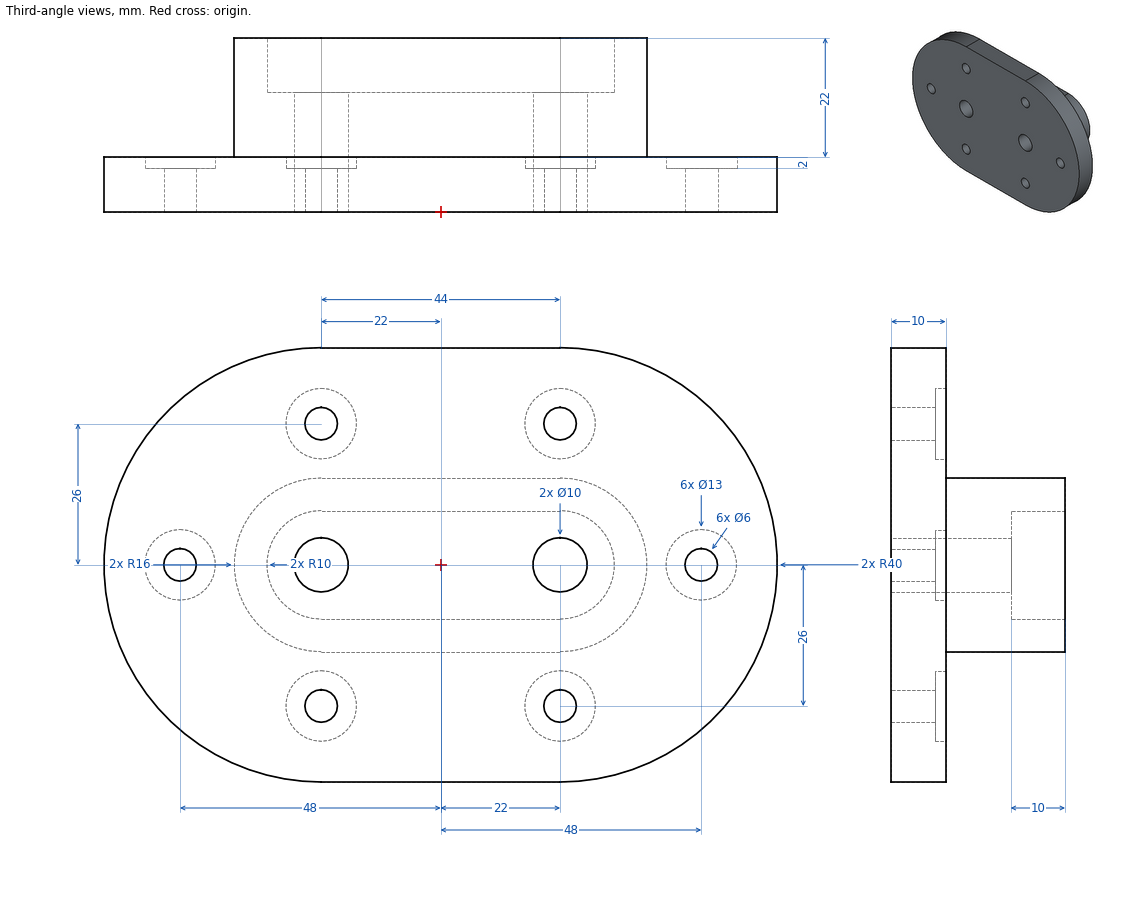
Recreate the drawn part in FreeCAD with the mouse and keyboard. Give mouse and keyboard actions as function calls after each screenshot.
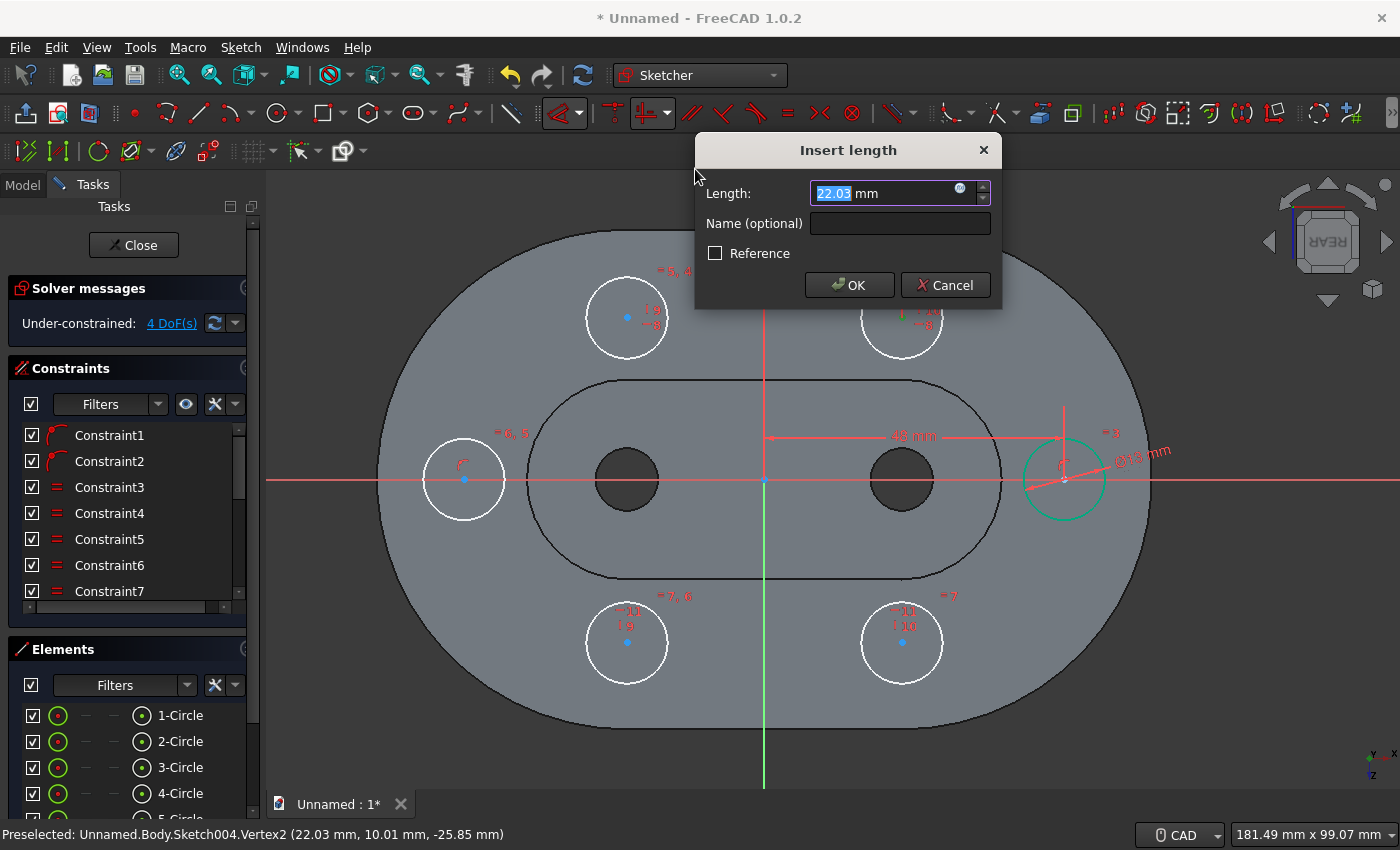
text(22)
key(Return)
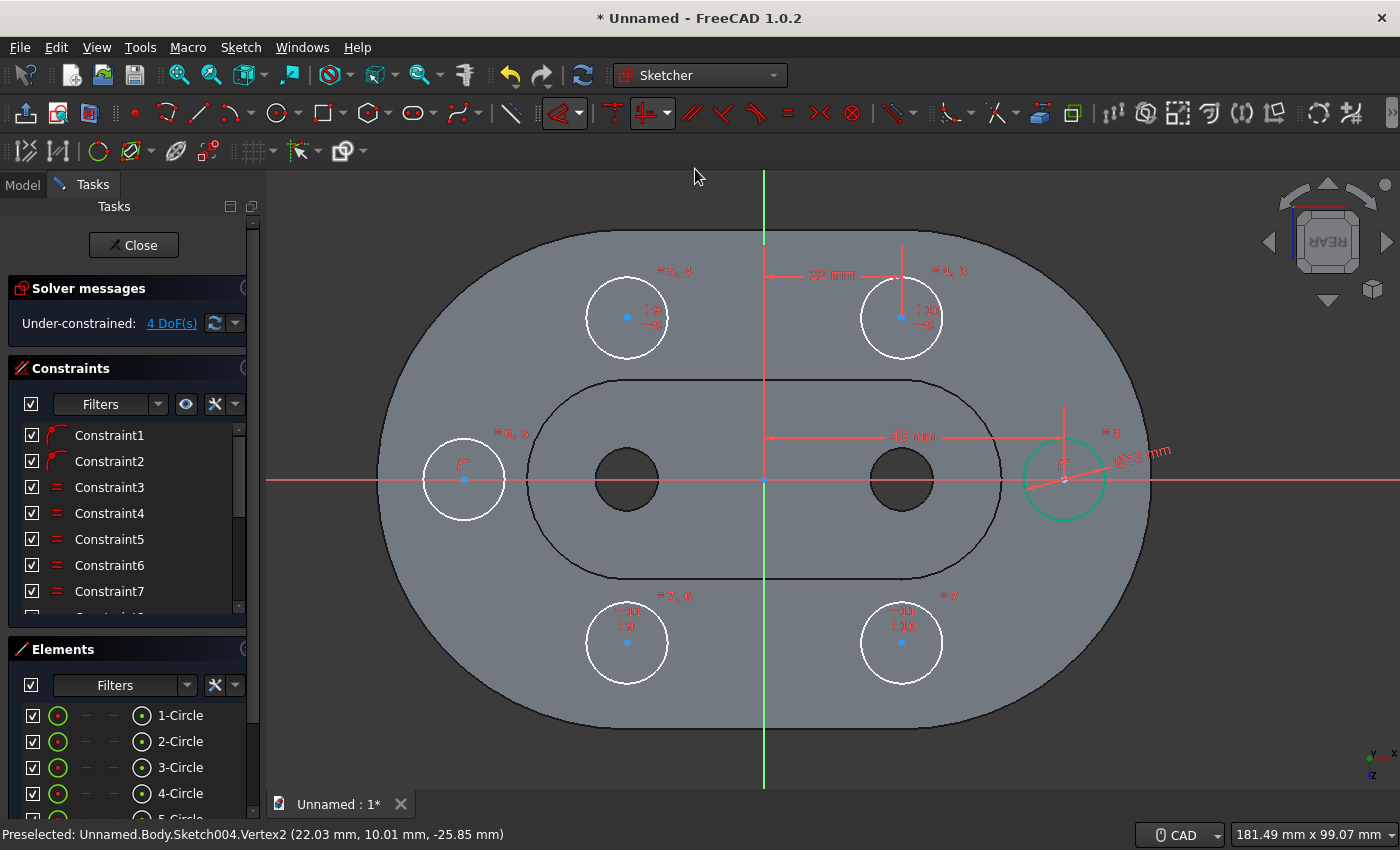
click(902, 318)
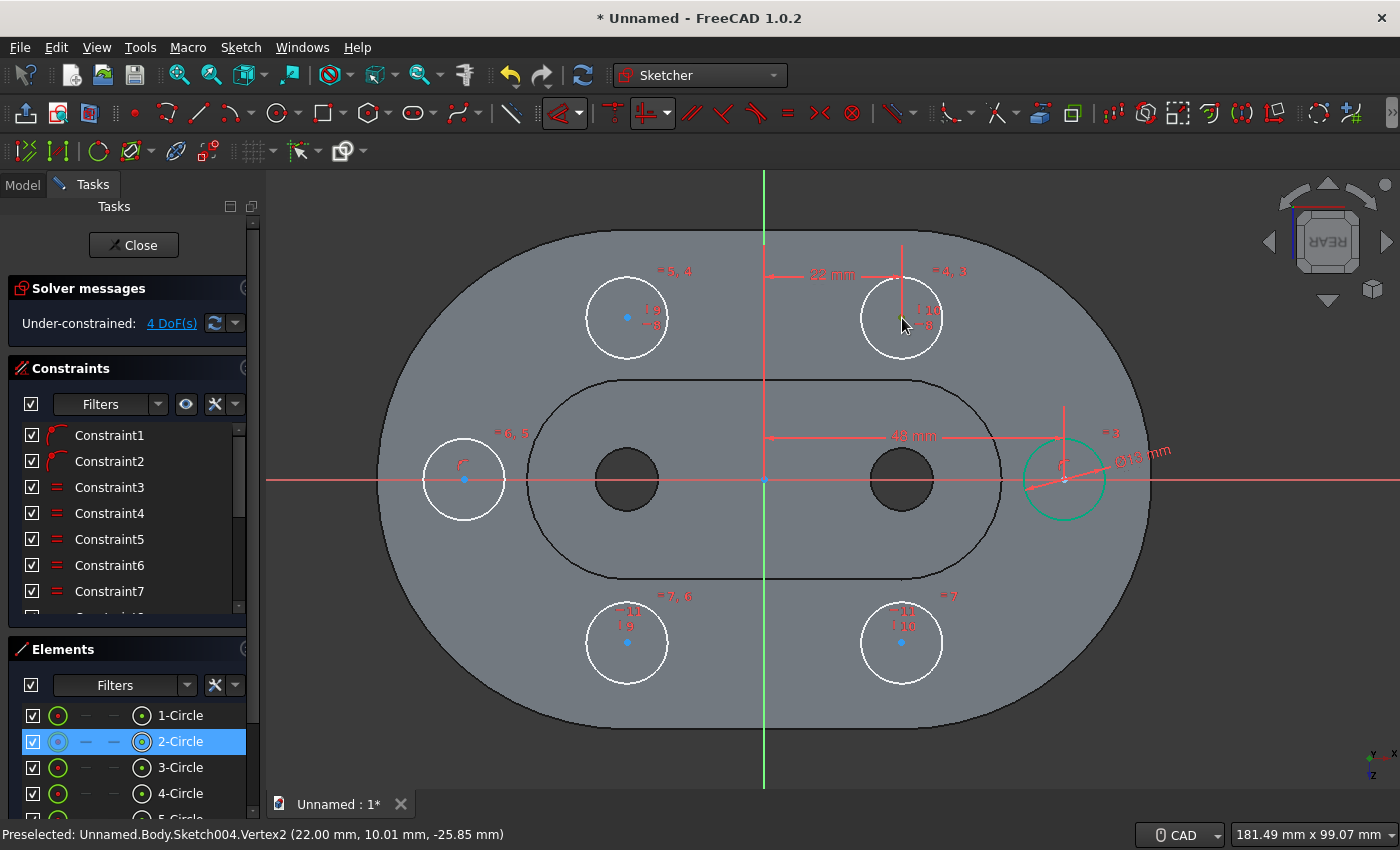
key(i)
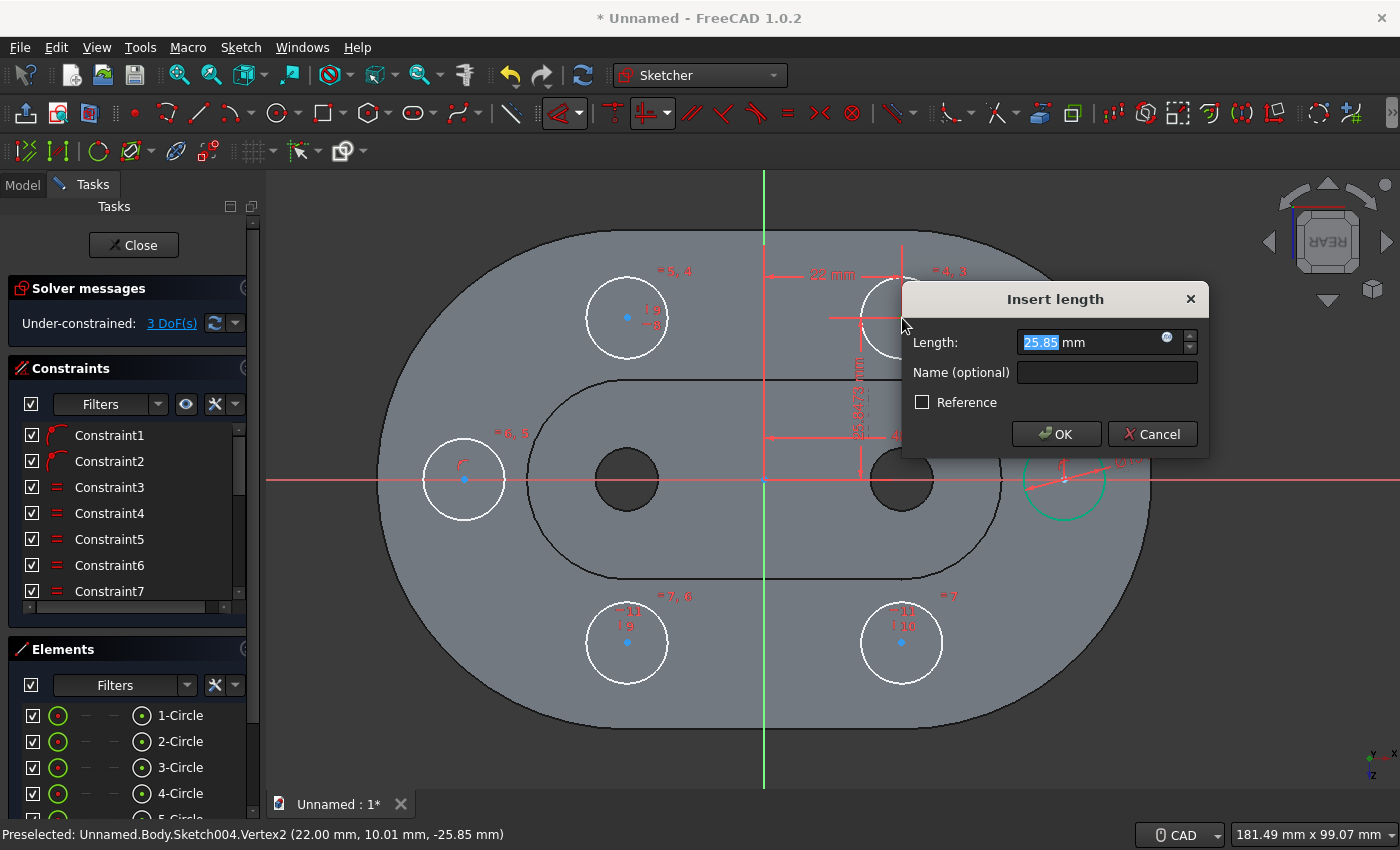
text(26)
key(Return)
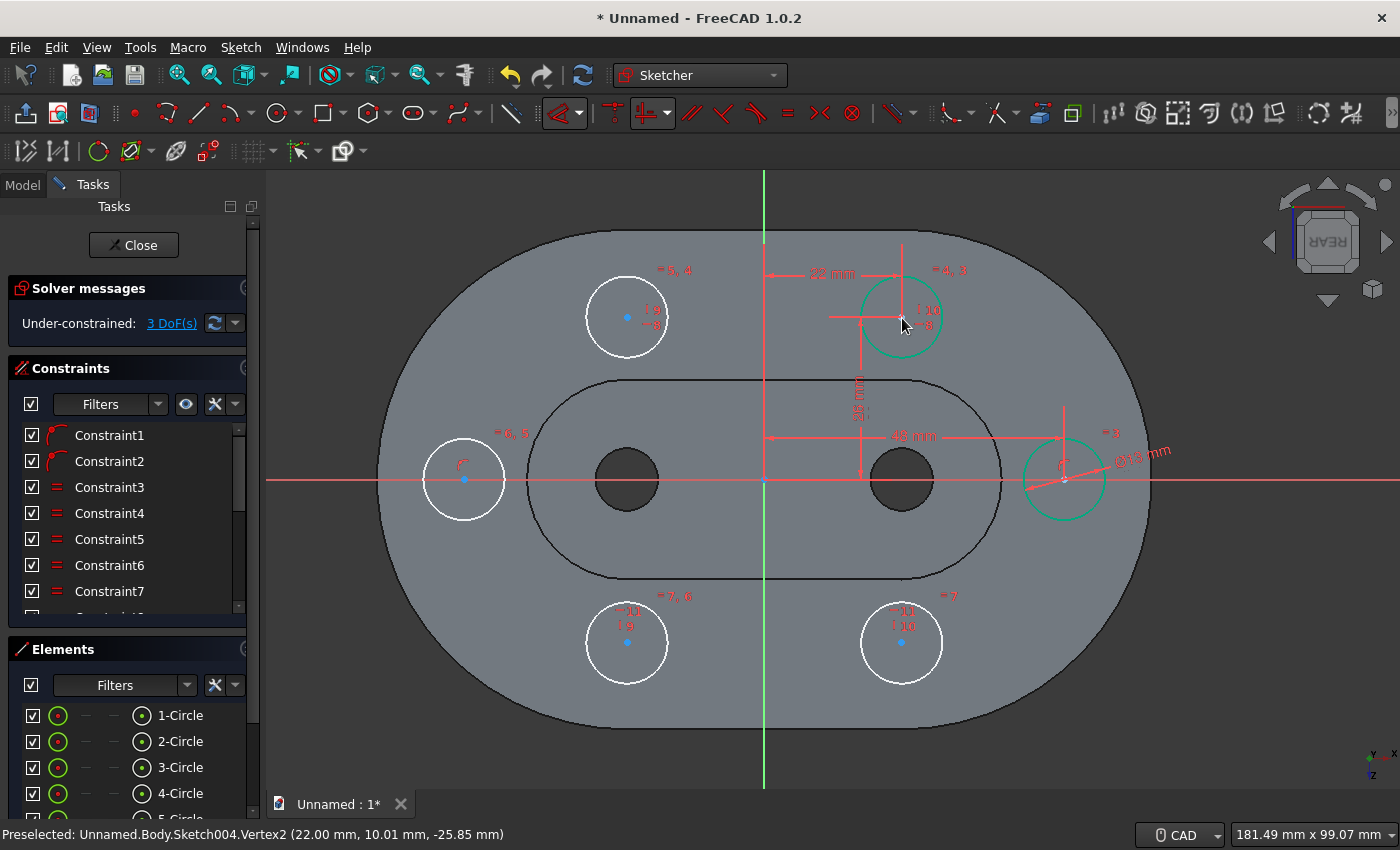
click(627, 317)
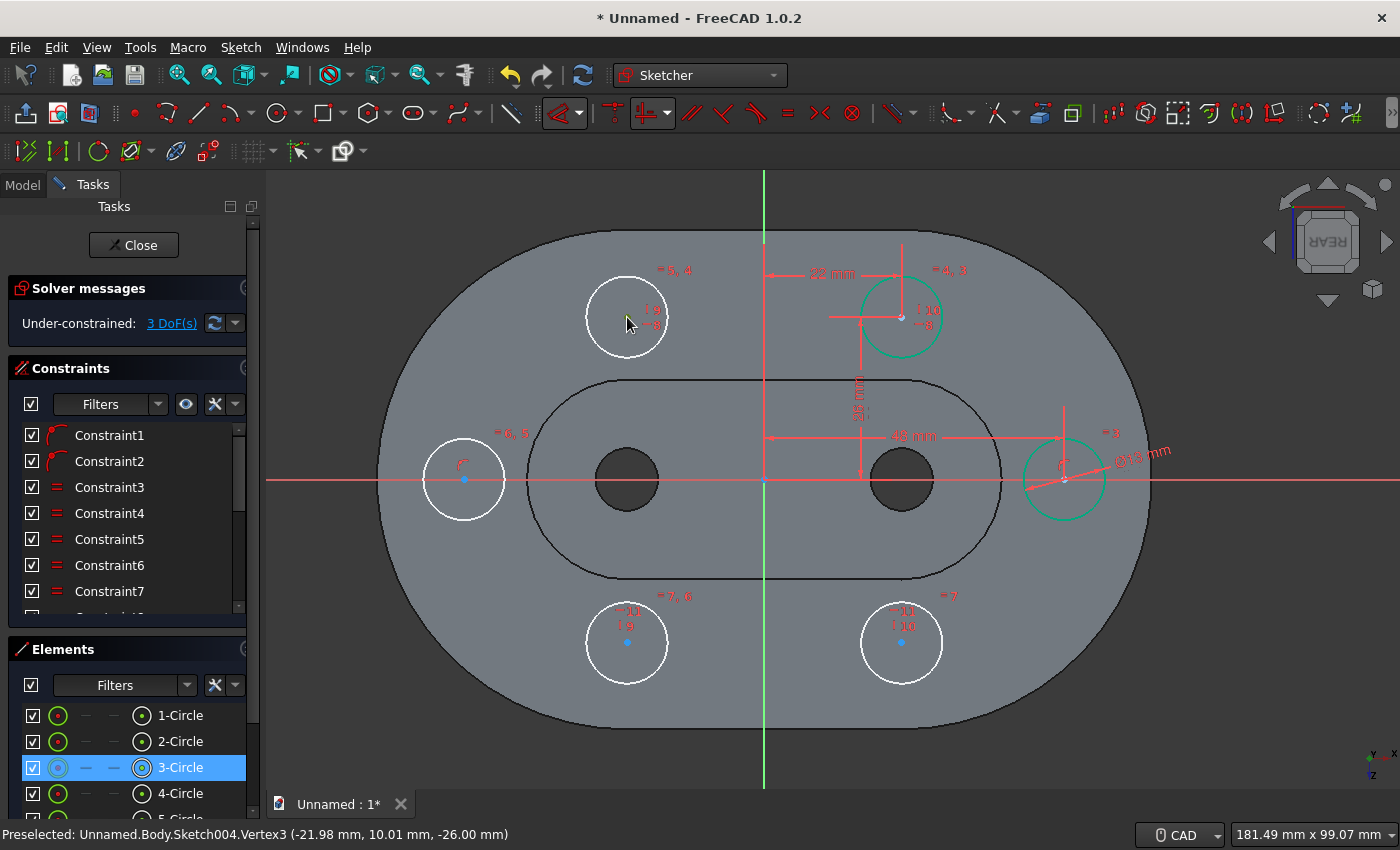
click(582, 114)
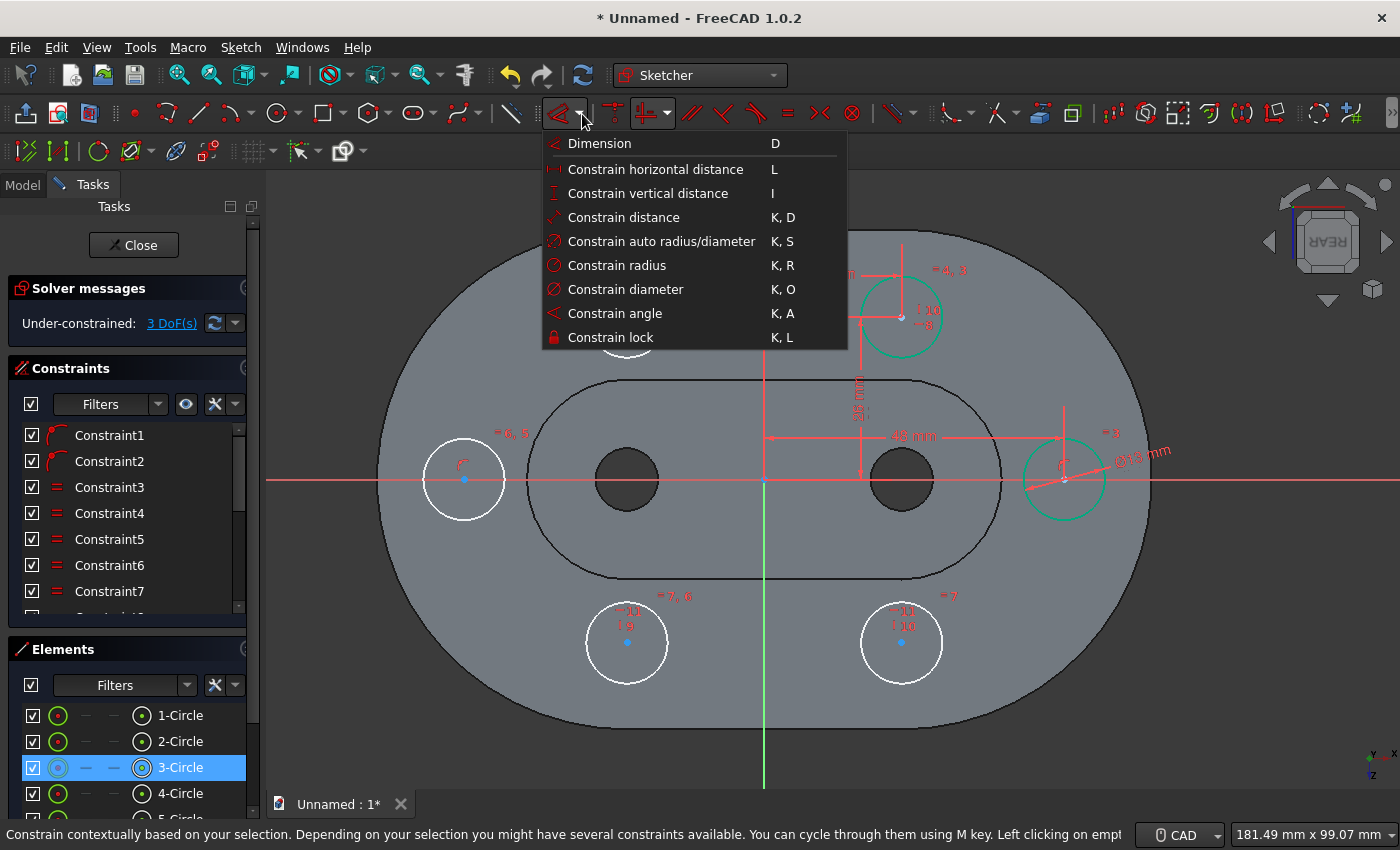
click(695, 169)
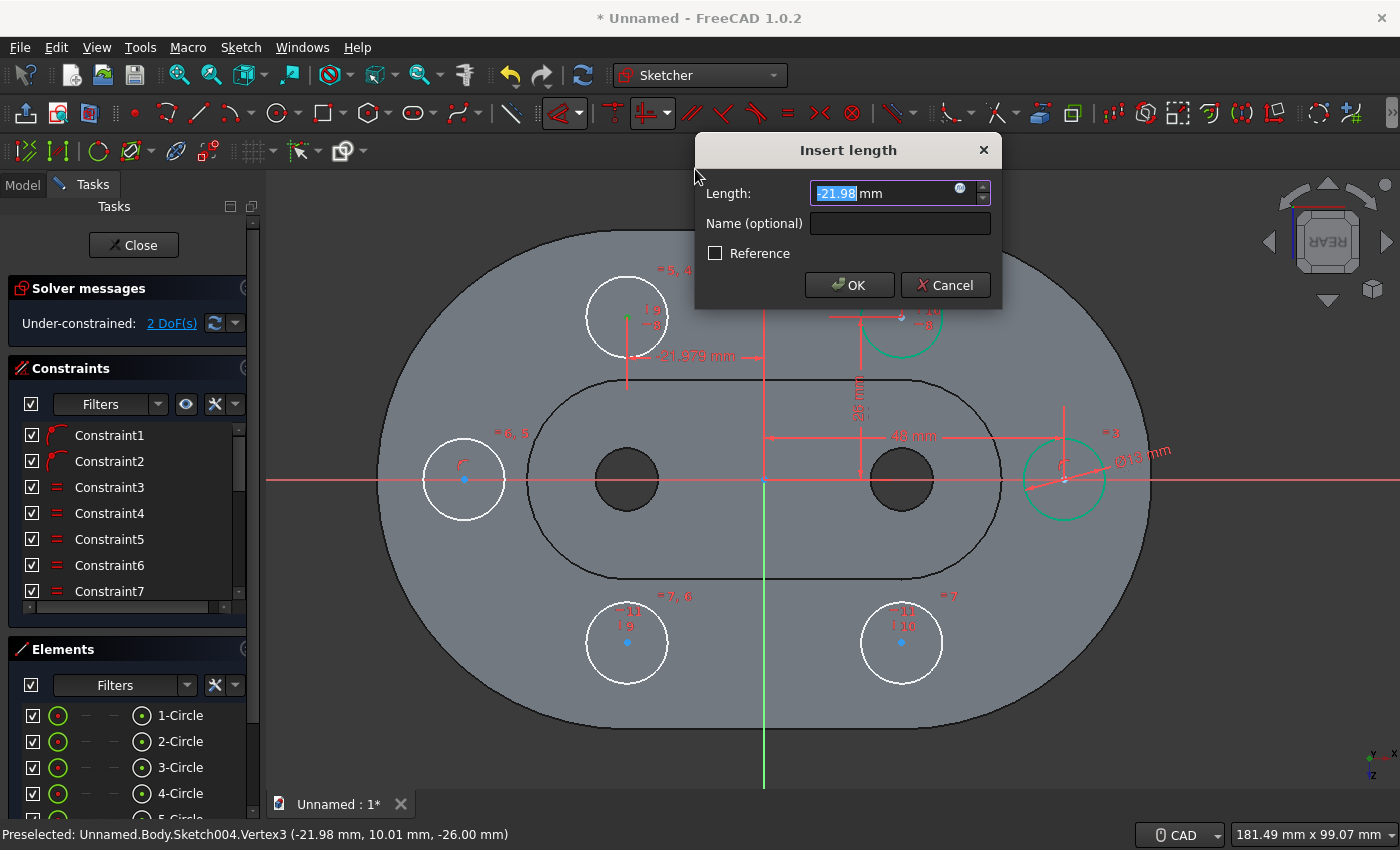
text(-22)
key(Return)